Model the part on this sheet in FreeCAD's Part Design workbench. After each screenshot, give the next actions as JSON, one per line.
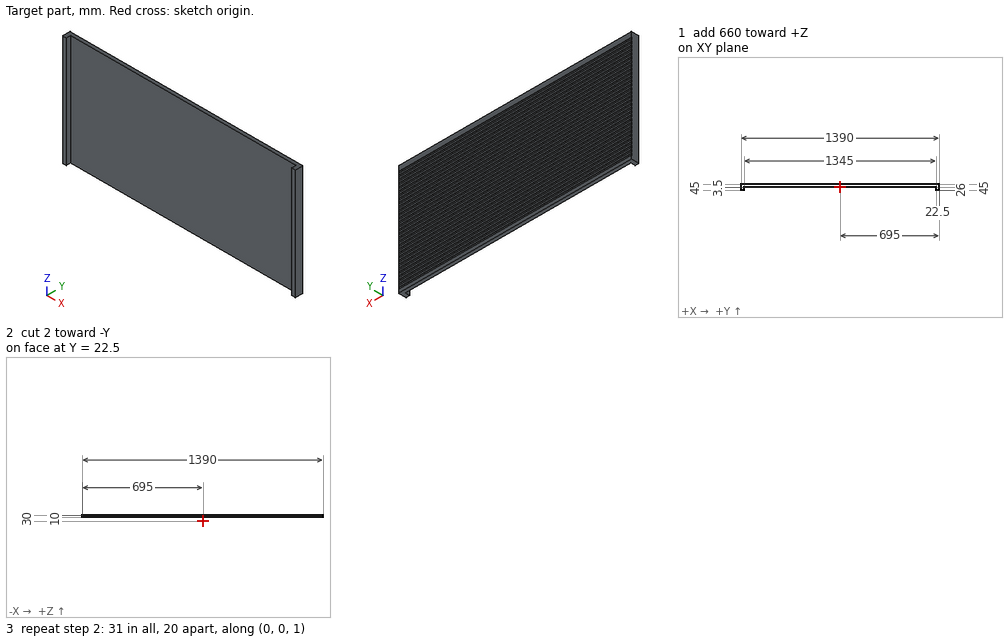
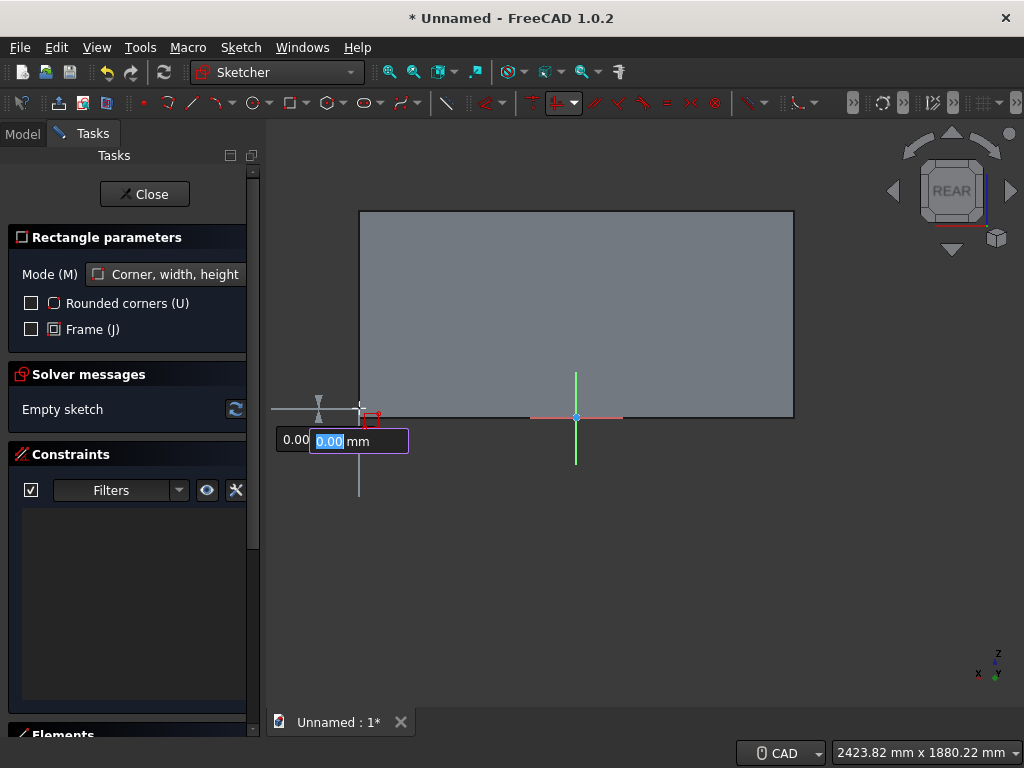
{"action": "scroll", "coordinate": [794, 412], "scroll_direction": "up", "scroll_amount": 5}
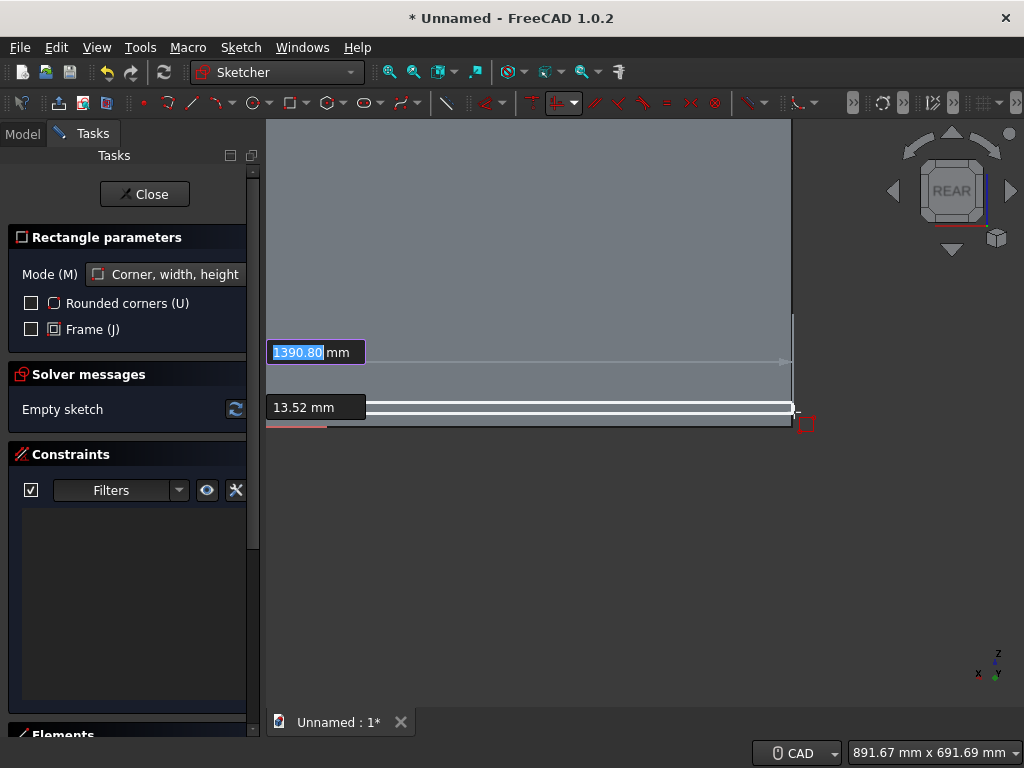
{"action": "left_click", "coordinate": [792, 410]}
{"action": "key", "text": "Escape"}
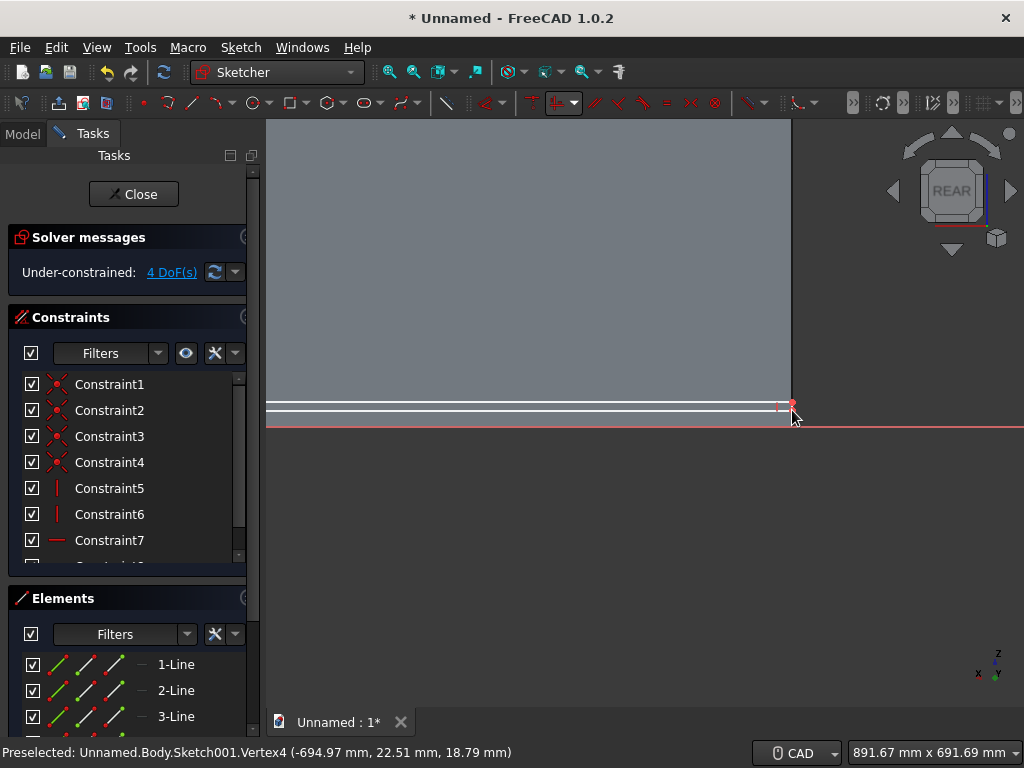
{"action": "key", "text": "d"}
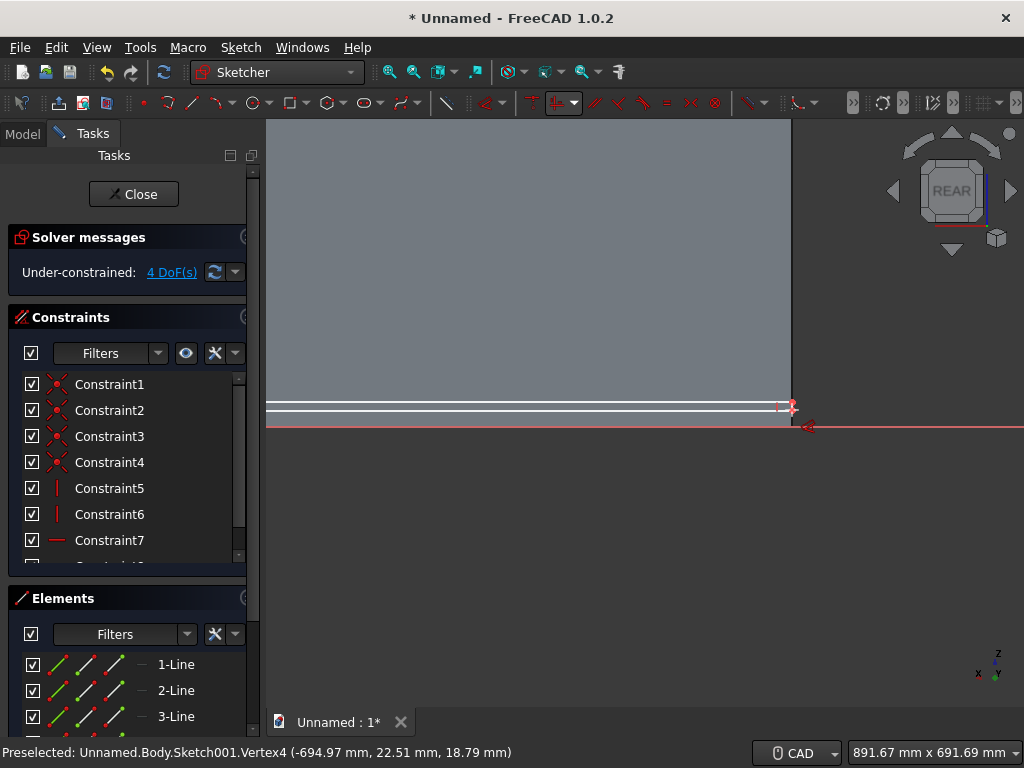
{"action": "scroll", "coordinate": [795, 412], "scroll_direction": "down", "scroll_amount": 5}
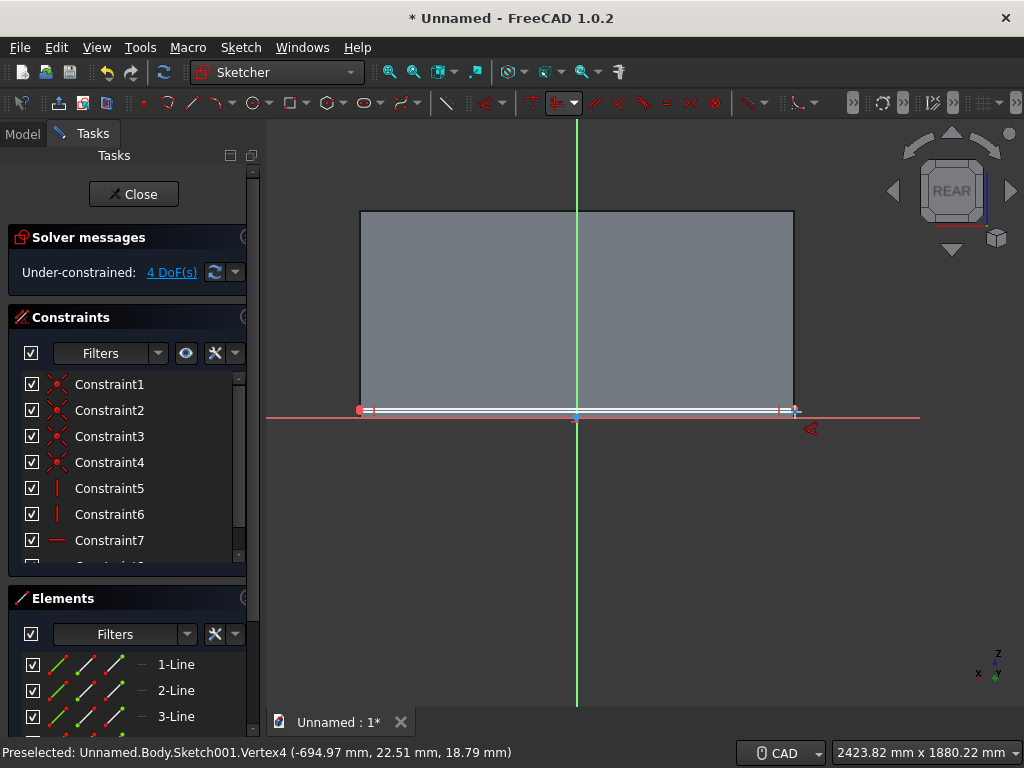
{"action": "scroll", "coordinate": [360, 410], "scroll_direction": "up", "scroll_amount": 13}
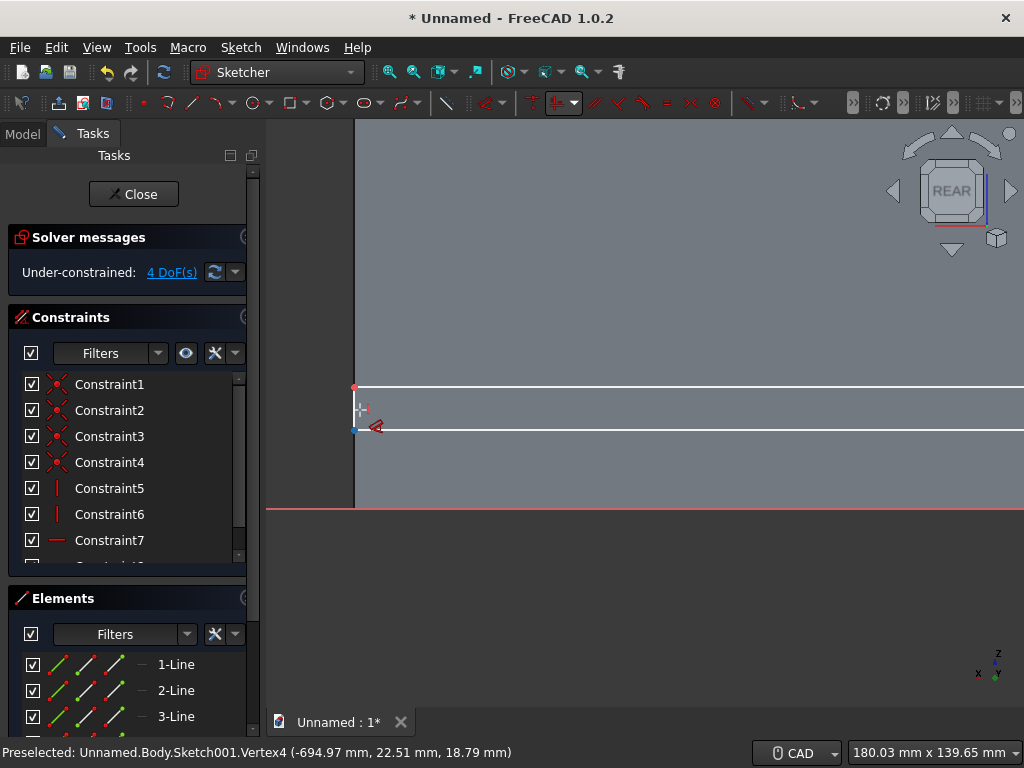
{"action": "left_click", "coordinate": [354, 409]}
{"action": "left_click", "coordinate": [320, 409]}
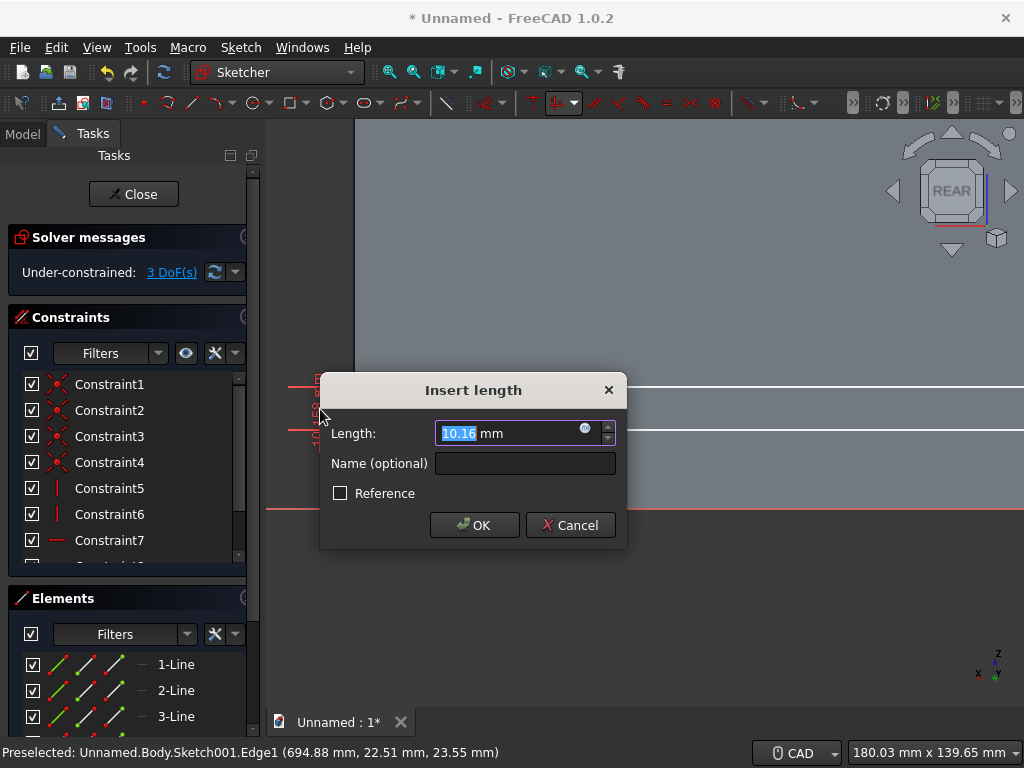
{"action": "type", "text": "10"}
{"action": "key", "text": "Return"}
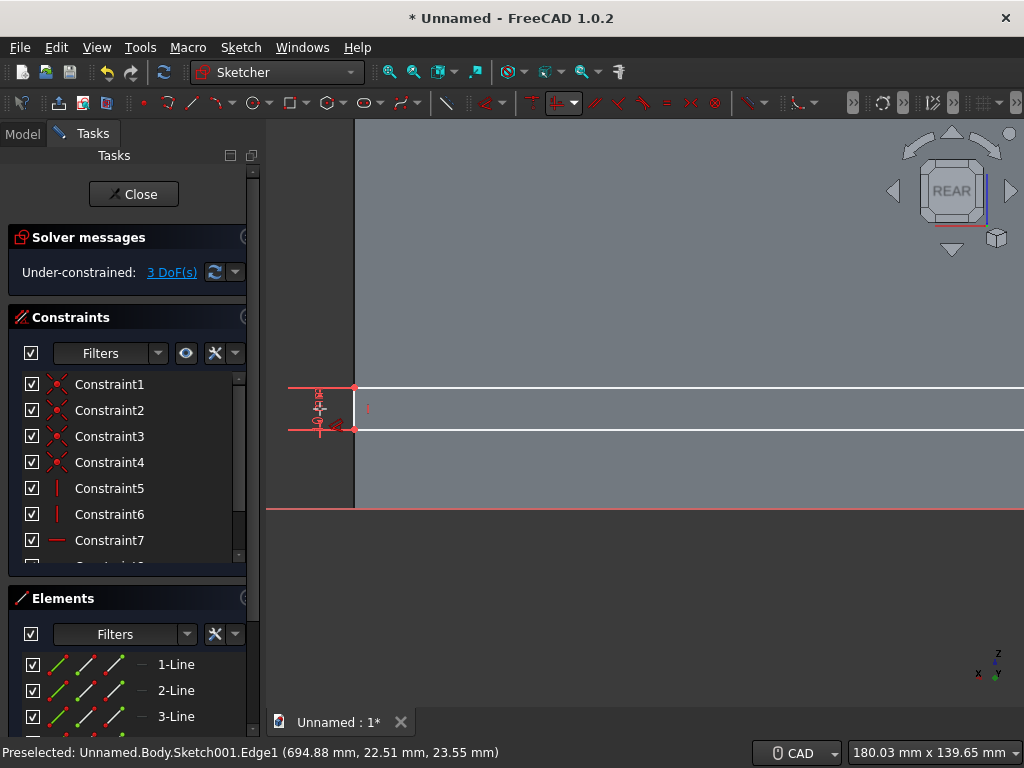
{"action": "scroll", "coordinate": [360, 410], "scroll_direction": "down", "scroll_amount": 13}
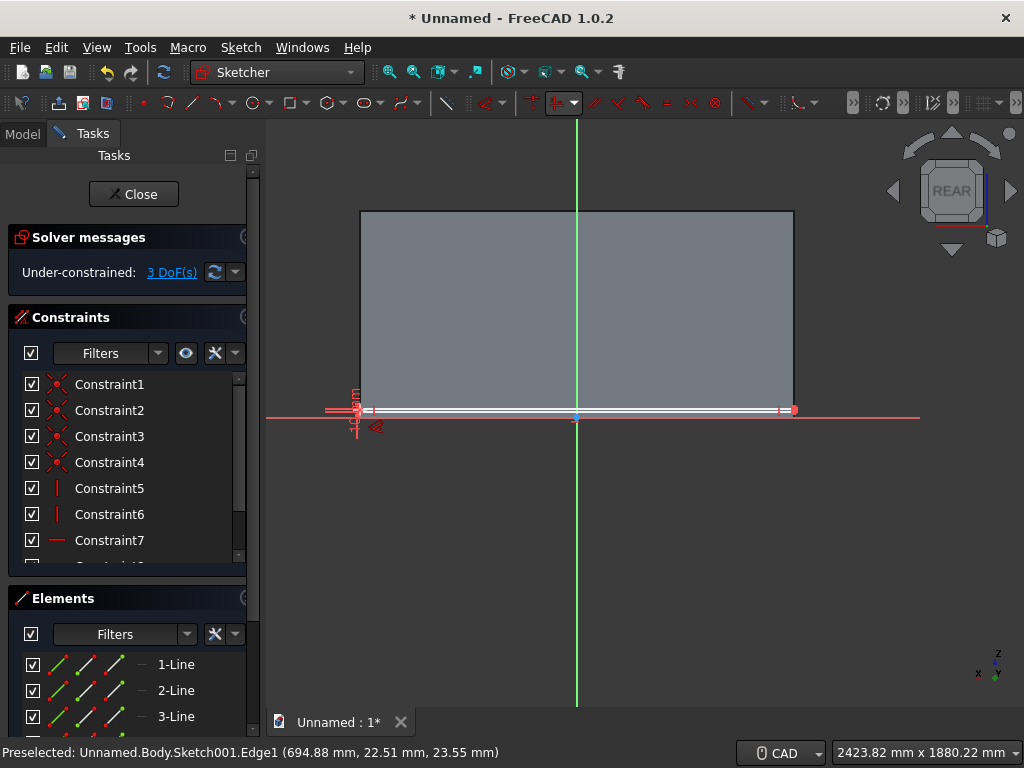
{"action": "scroll", "coordinate": [360, 409], "scroll_direction": "up", "scroll_amount": 8}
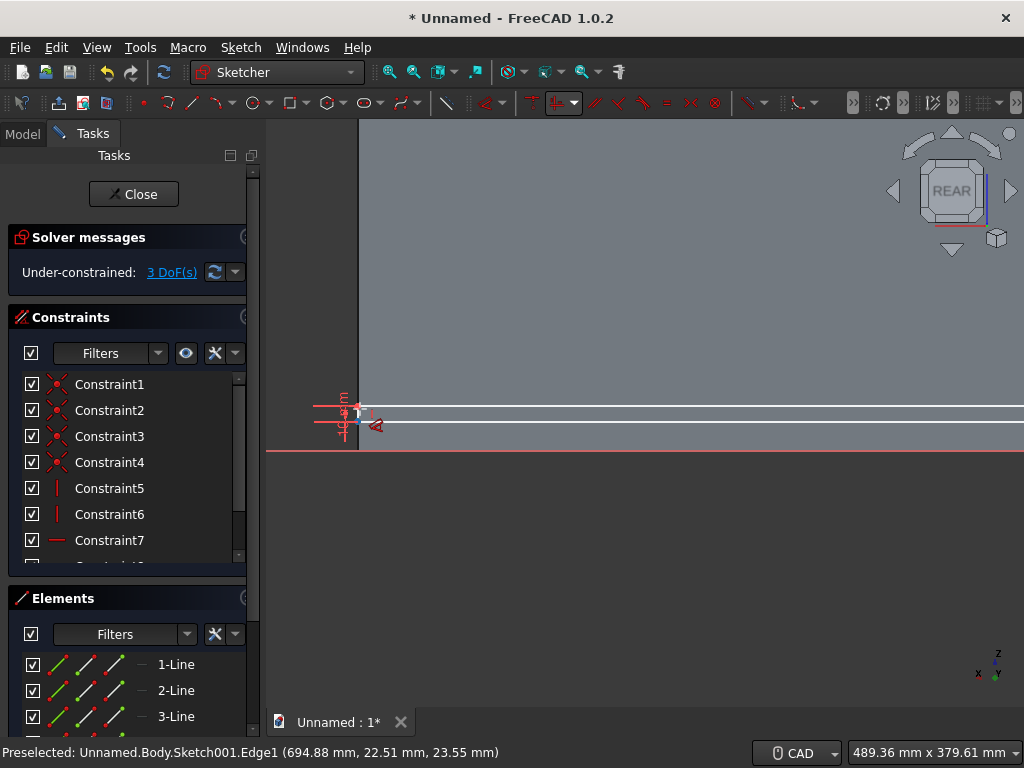
{"action": "left_click", "coordinate": [358, 406]}
{"action": "left_click", "coordinate": [324, 428]}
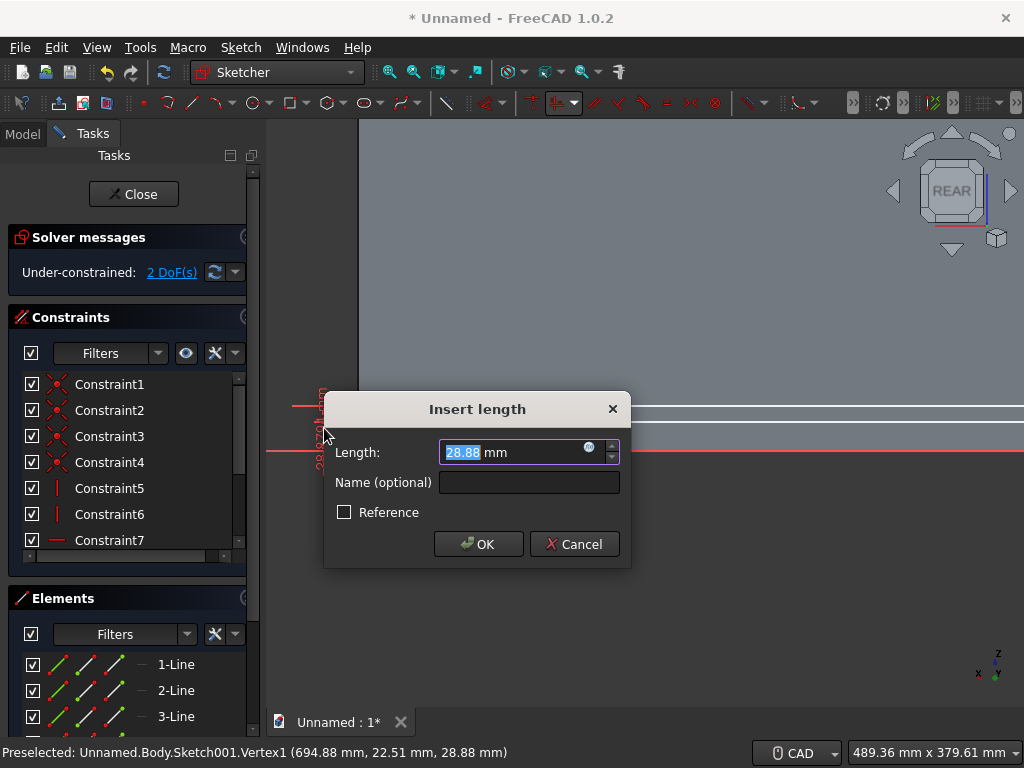
{"action": "type", "text": "30"}
{"action": "key", "text": "Return"}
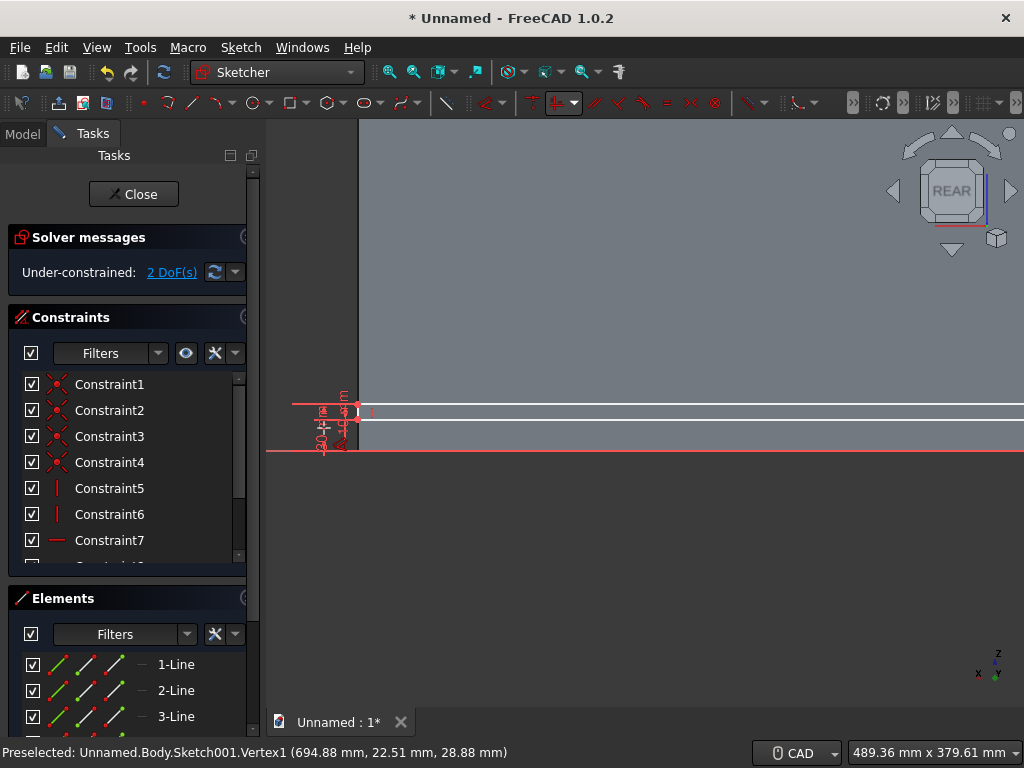
{"action": "left_click", "coordinate": [789, 420]}
{"action": "left_click", "coordinate": [608, 386]}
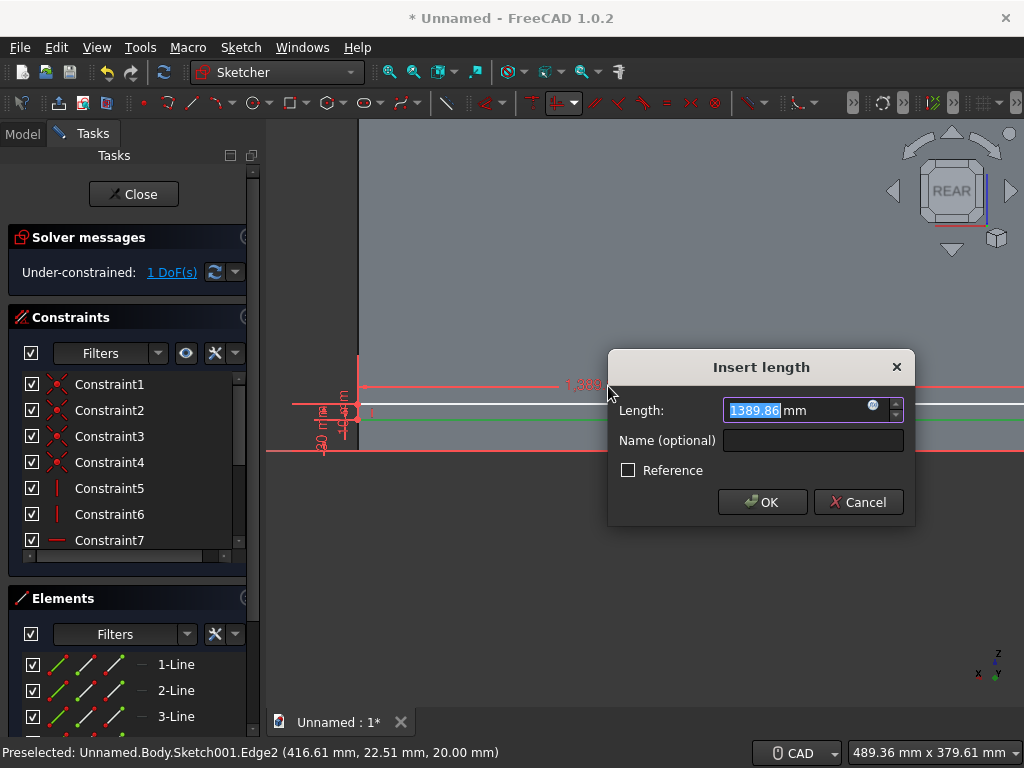
{"action": "type", "text": "1390"}
{"action": "key", "text": "Return"}